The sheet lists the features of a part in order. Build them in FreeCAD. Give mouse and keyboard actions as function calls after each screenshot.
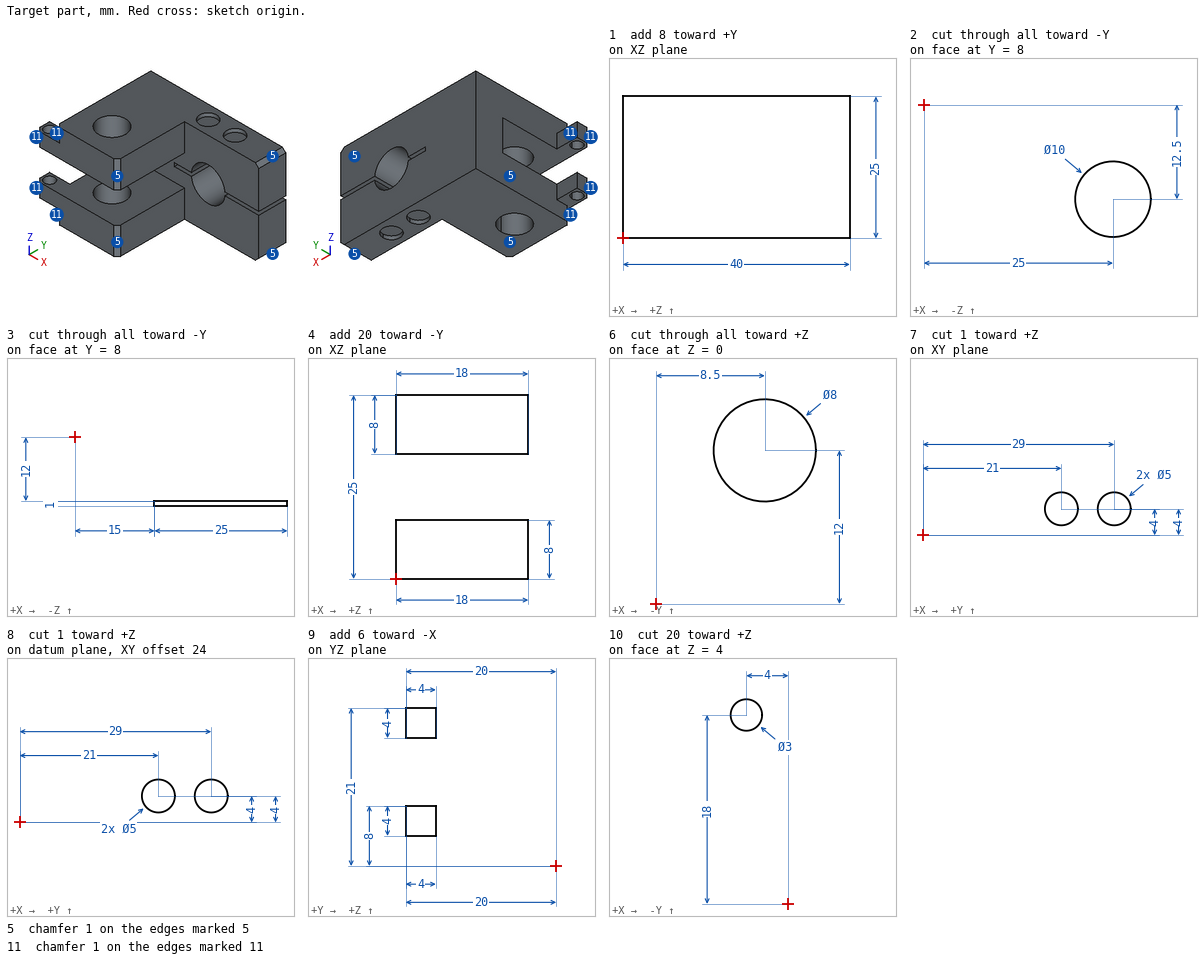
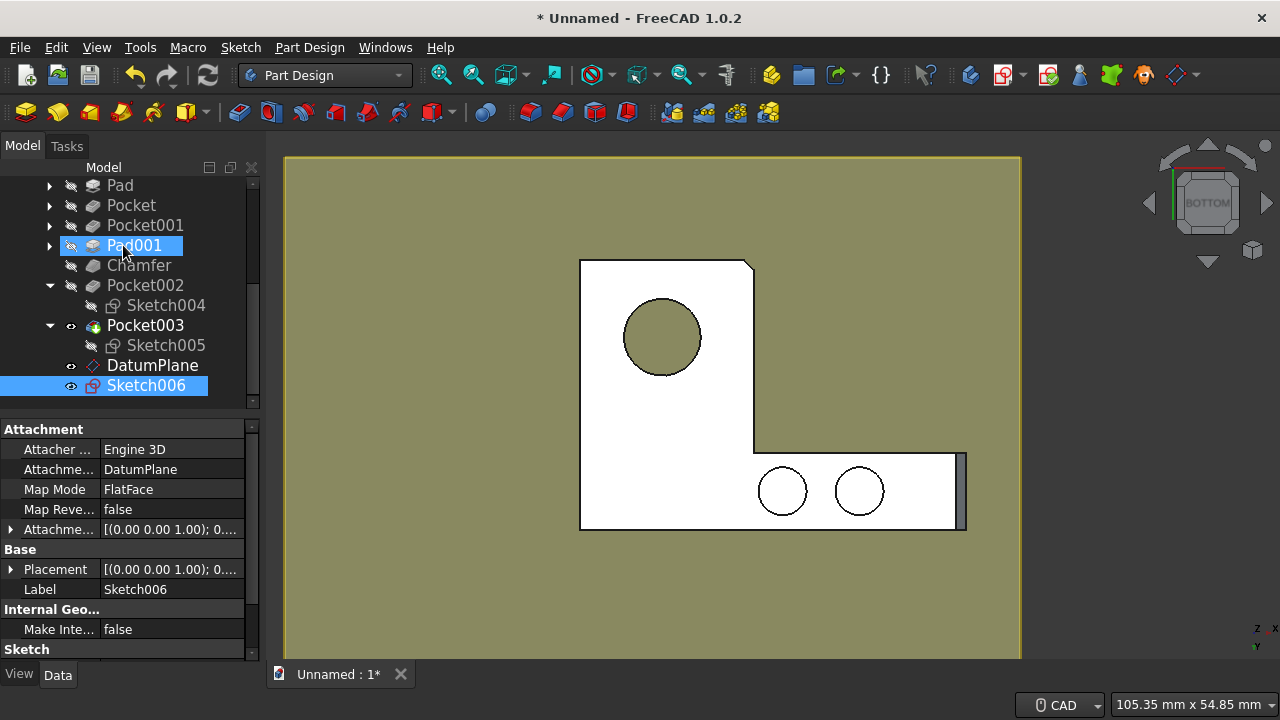
click(240, 112)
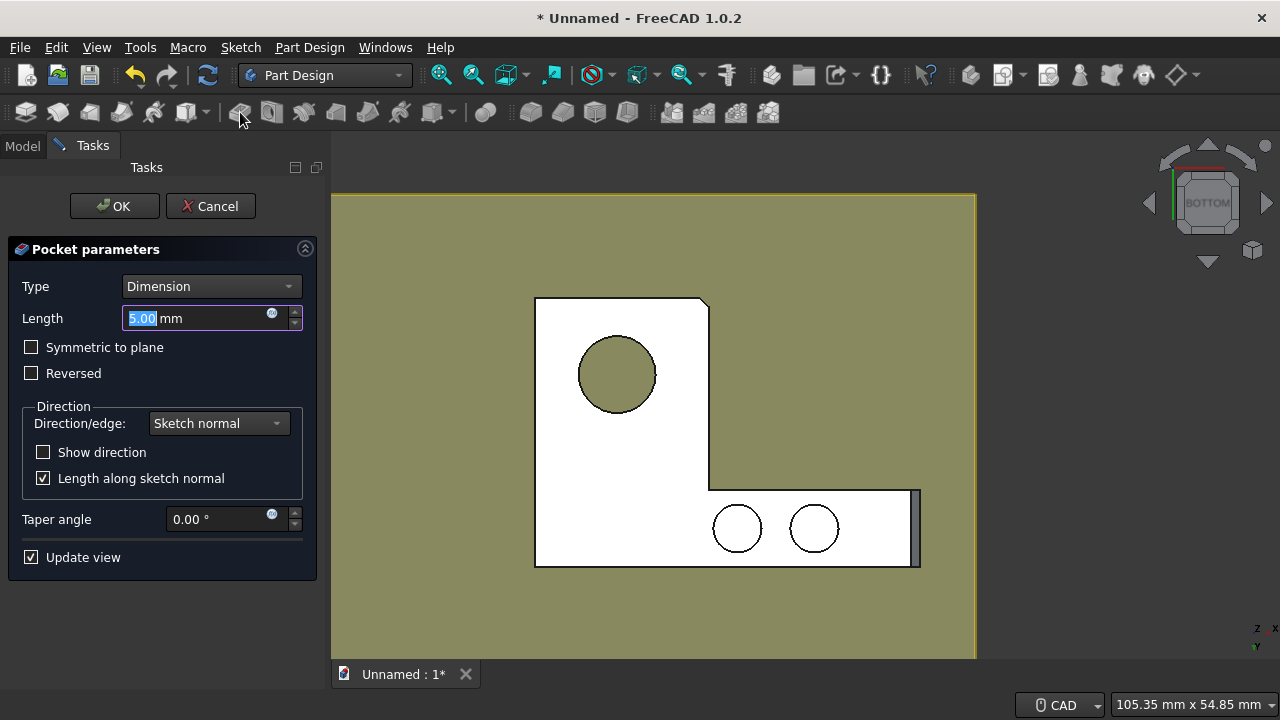
text(1)
key(Tab)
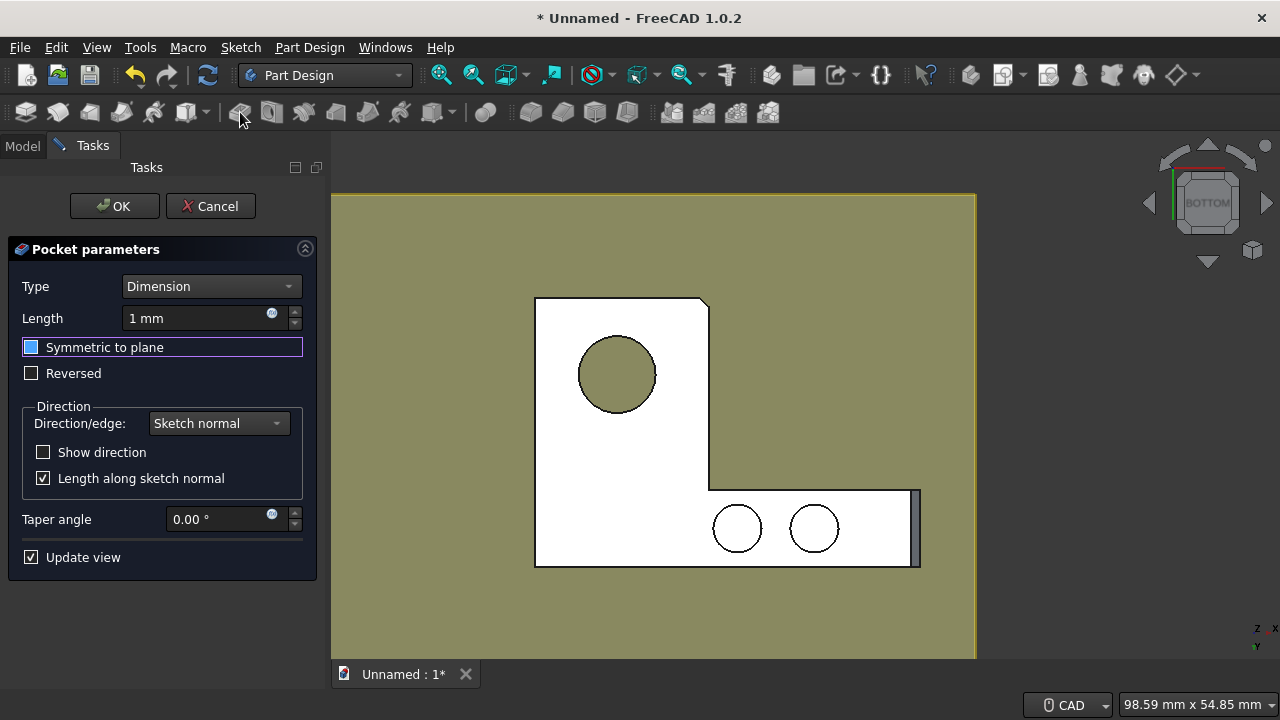
click(30, 373)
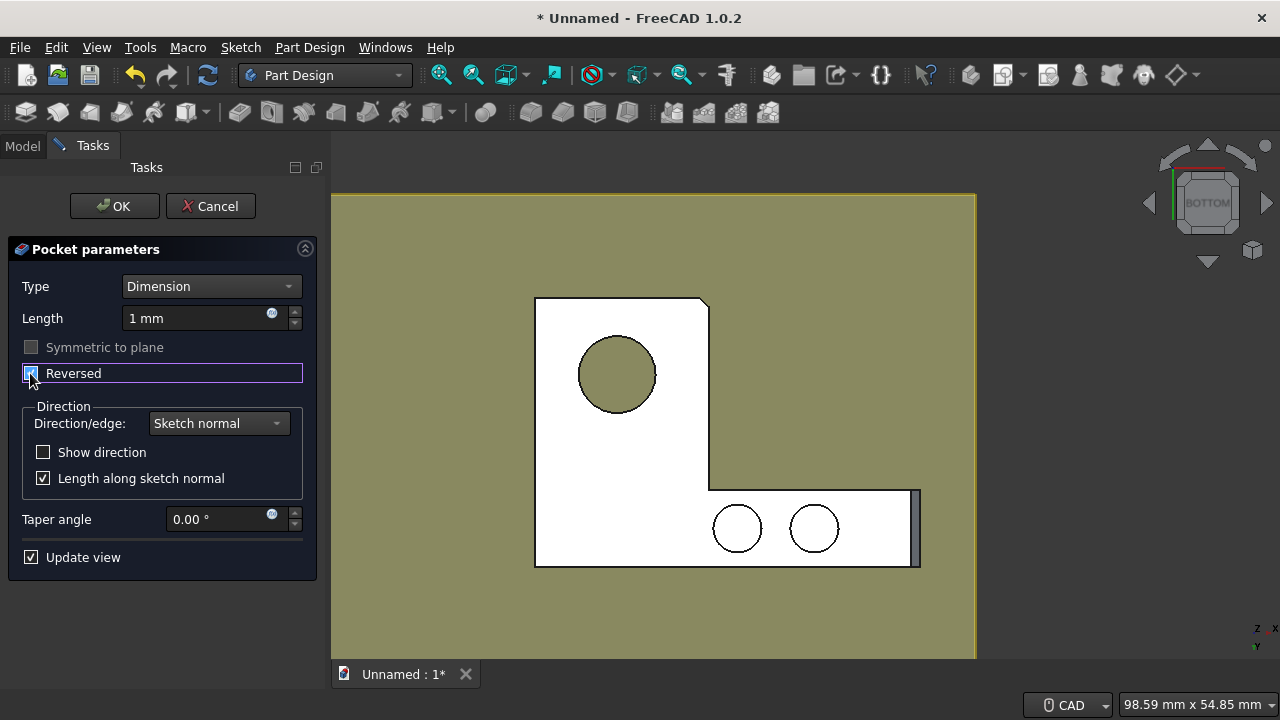
click(115, 206)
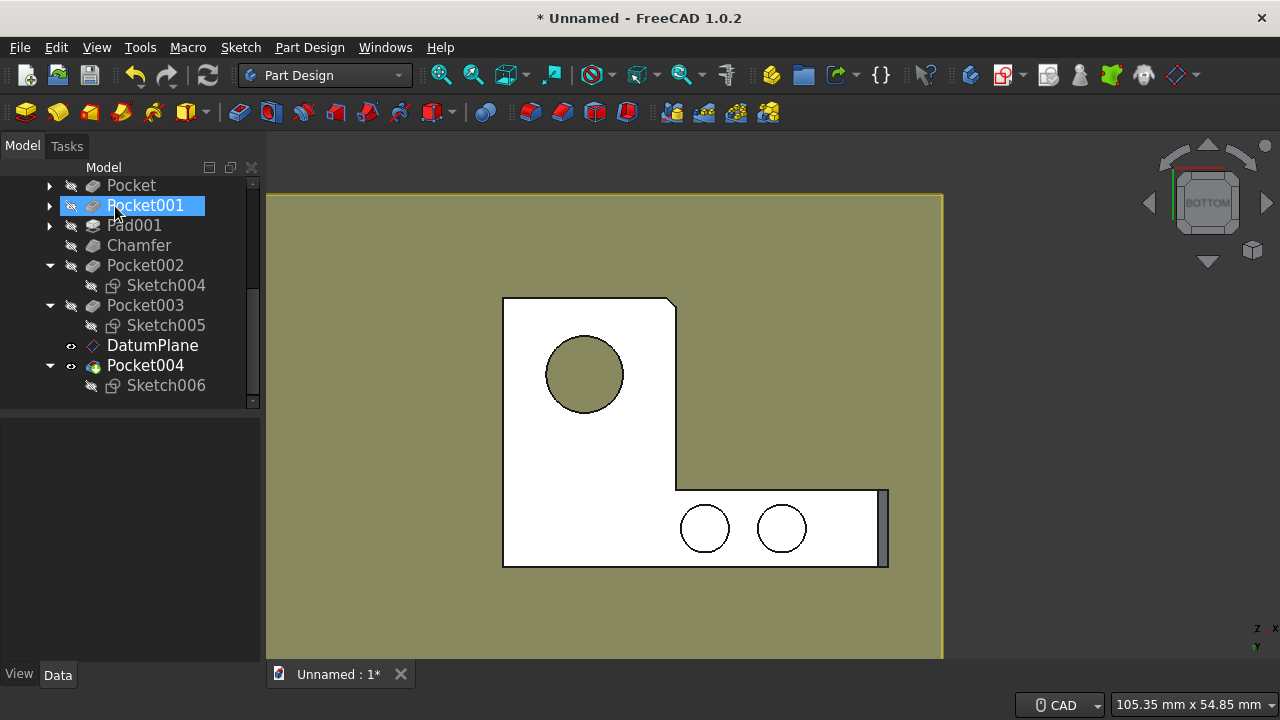
click(116, 346)
key(space)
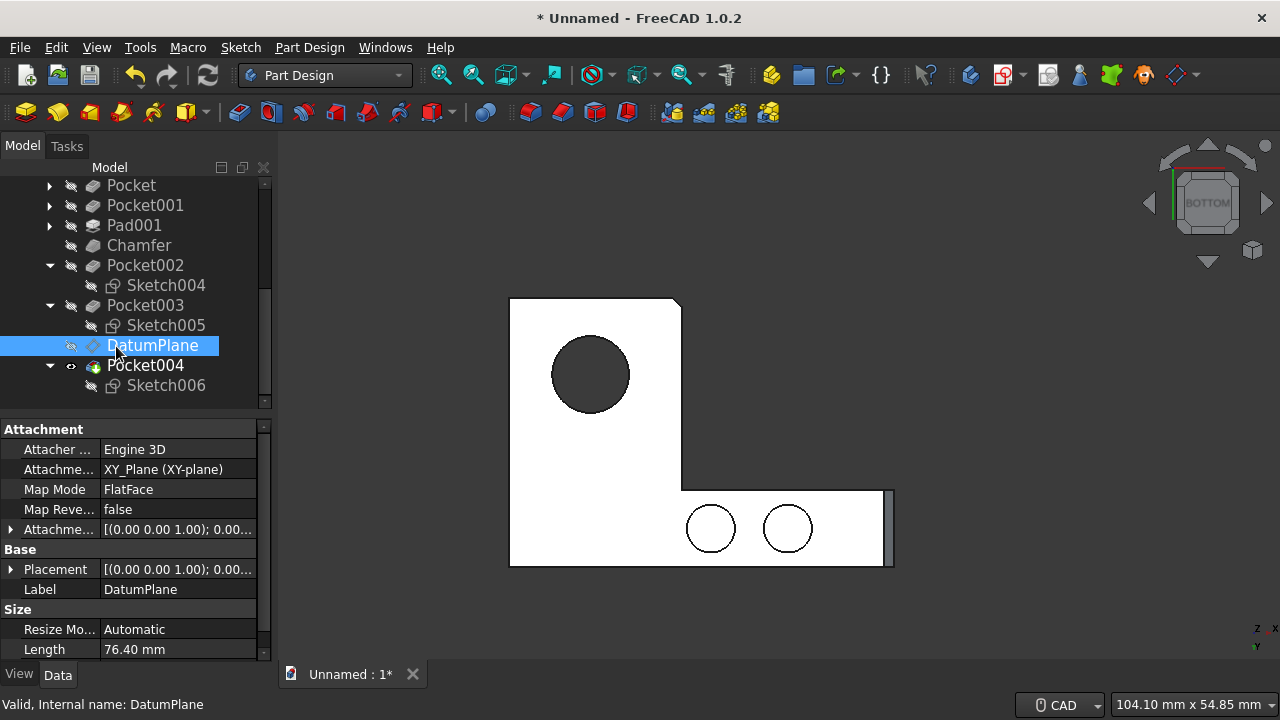
click(318, 619)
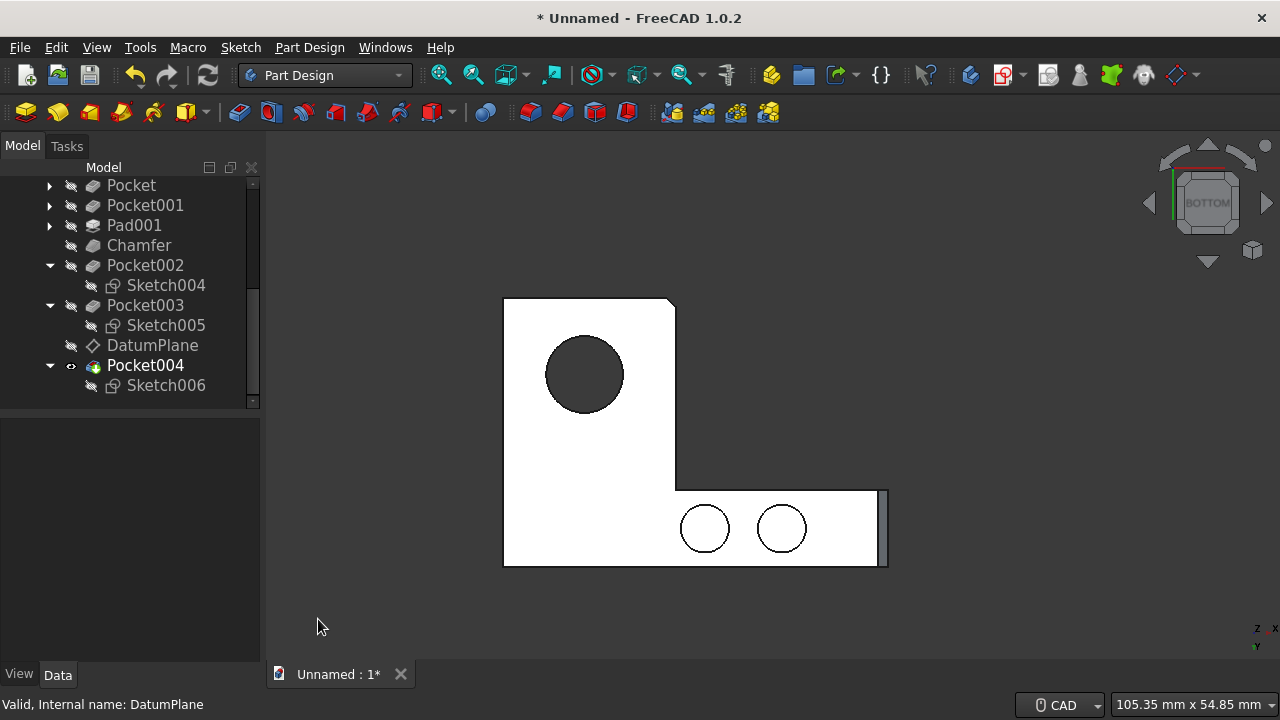
click(1004, 76)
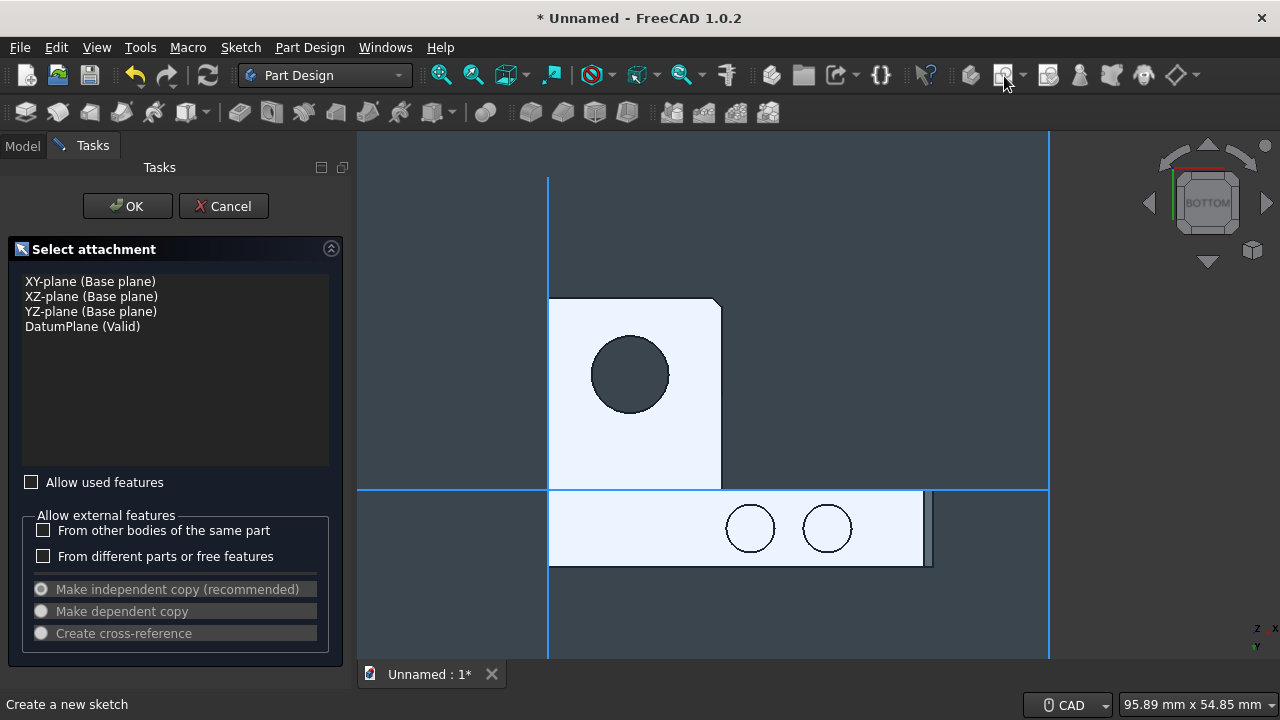
click(82, 312)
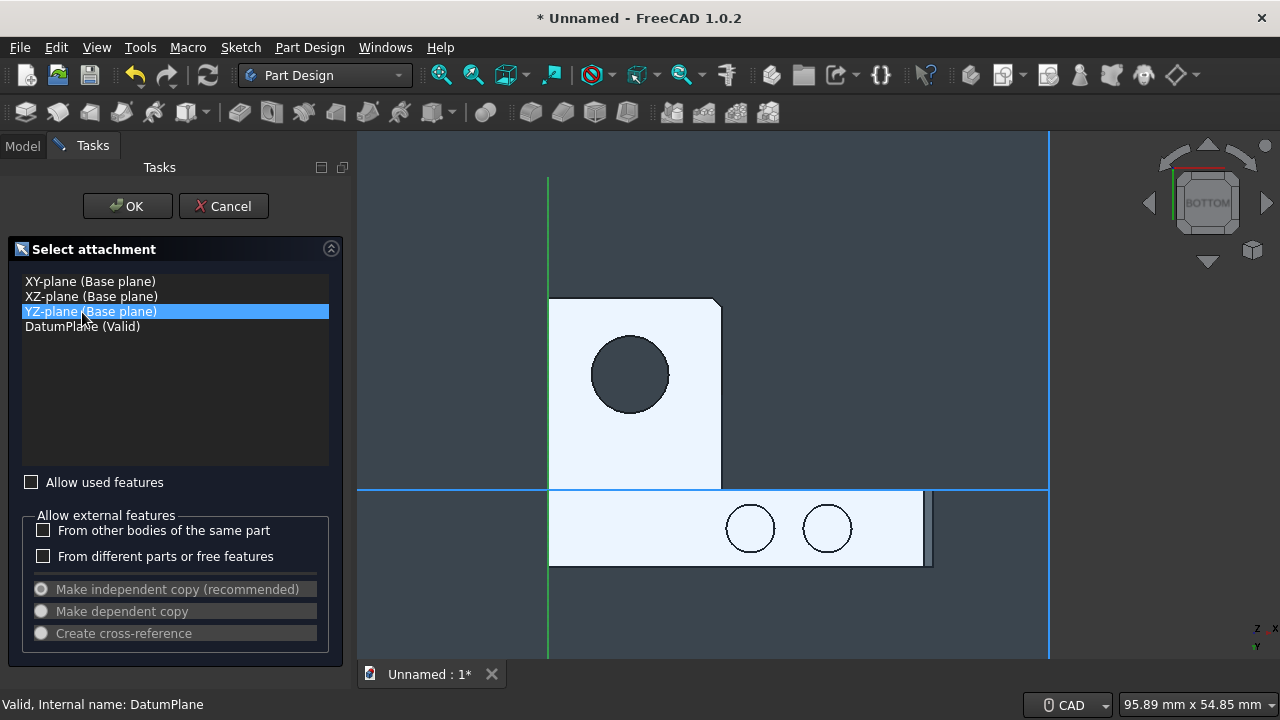
click(128, 206)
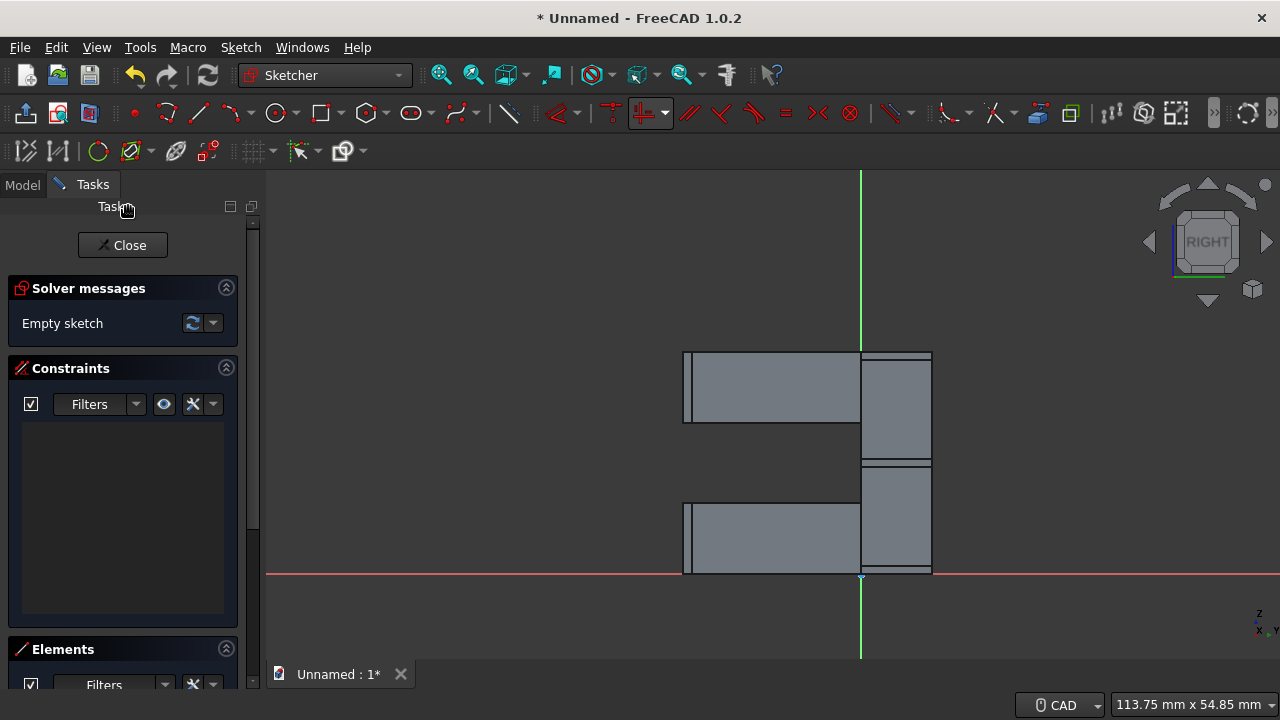
click(90, 114)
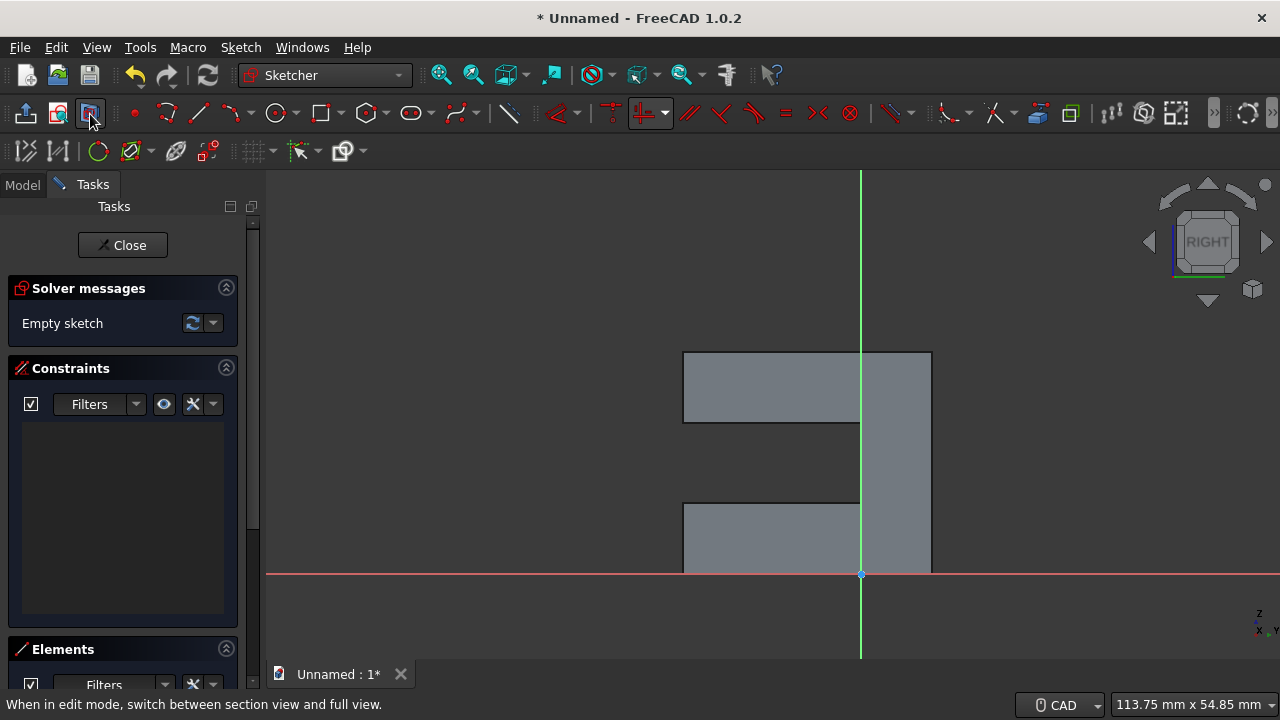
scroll(909, 616, up, 2)